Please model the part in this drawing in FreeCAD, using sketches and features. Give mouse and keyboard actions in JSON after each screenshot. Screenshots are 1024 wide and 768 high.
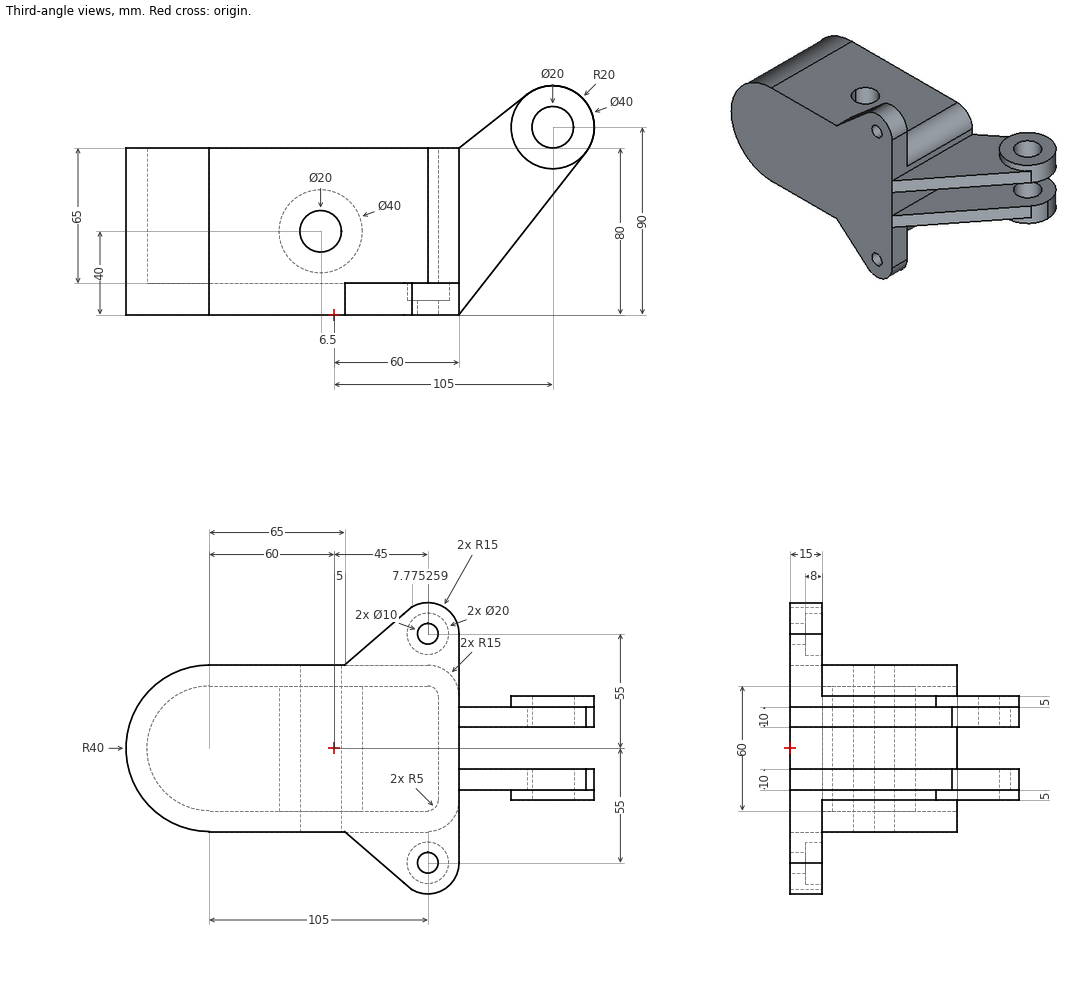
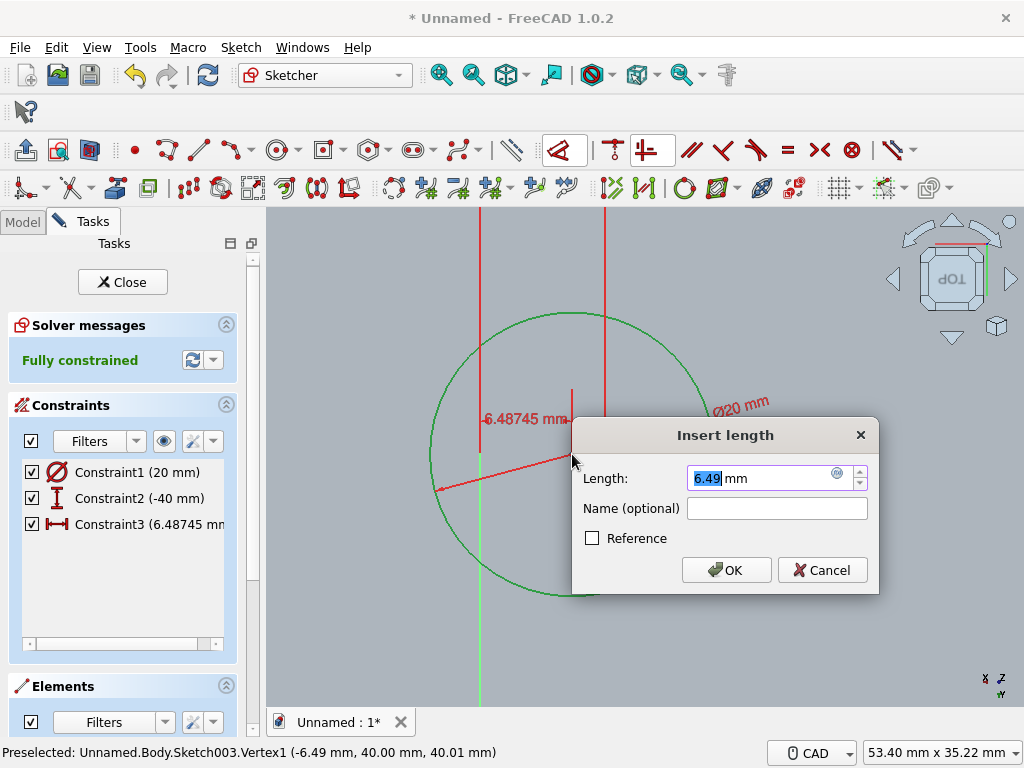
{"action": "type", "text": "6.5"}
{"action": "key", "text": "Return"}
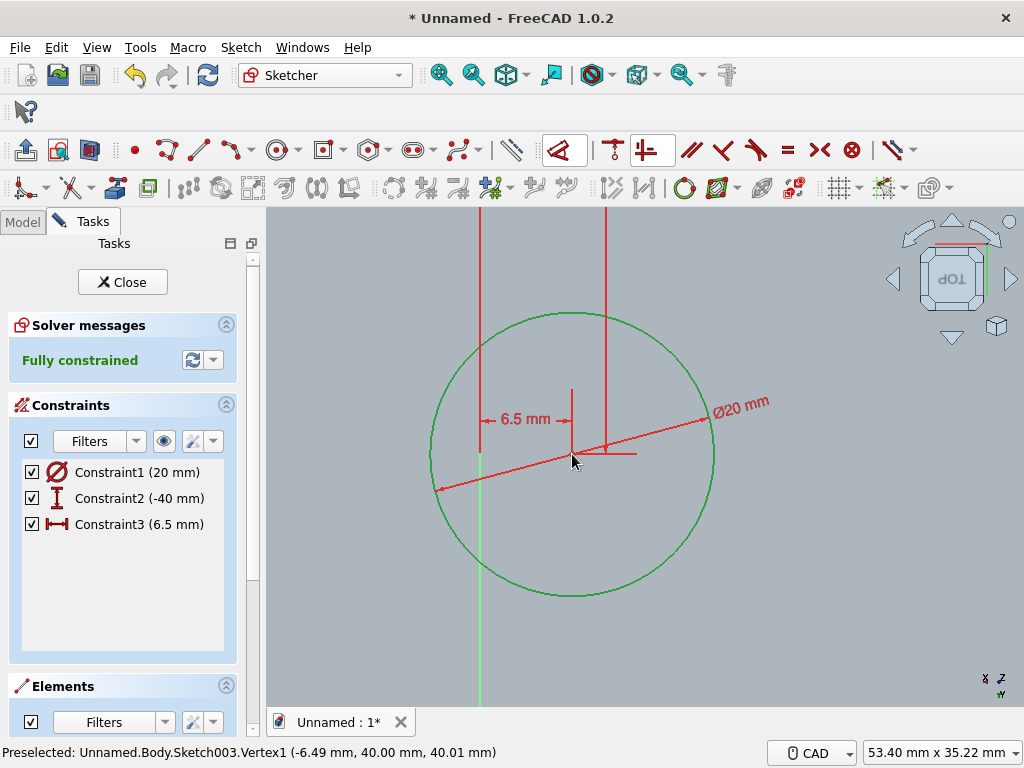
{"action": "left_click", "coordinate": [123, 282]}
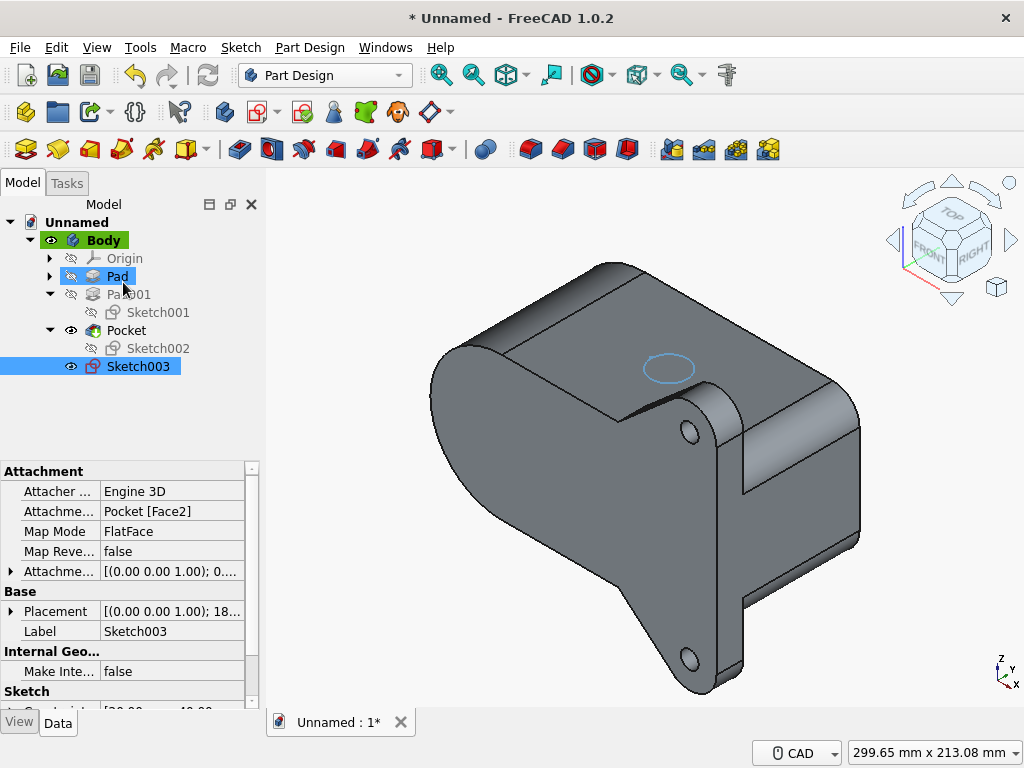
{"action": "left_click", "coordinate": [240, 150]}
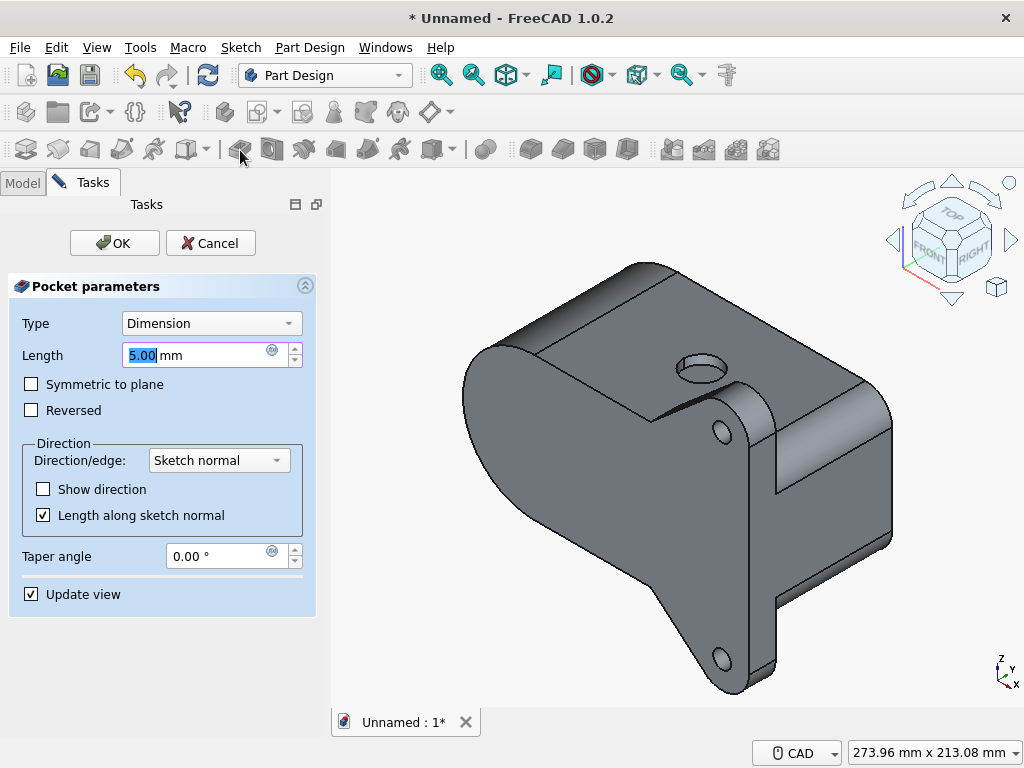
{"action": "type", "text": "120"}
{"action": "key", "text": "Tab"}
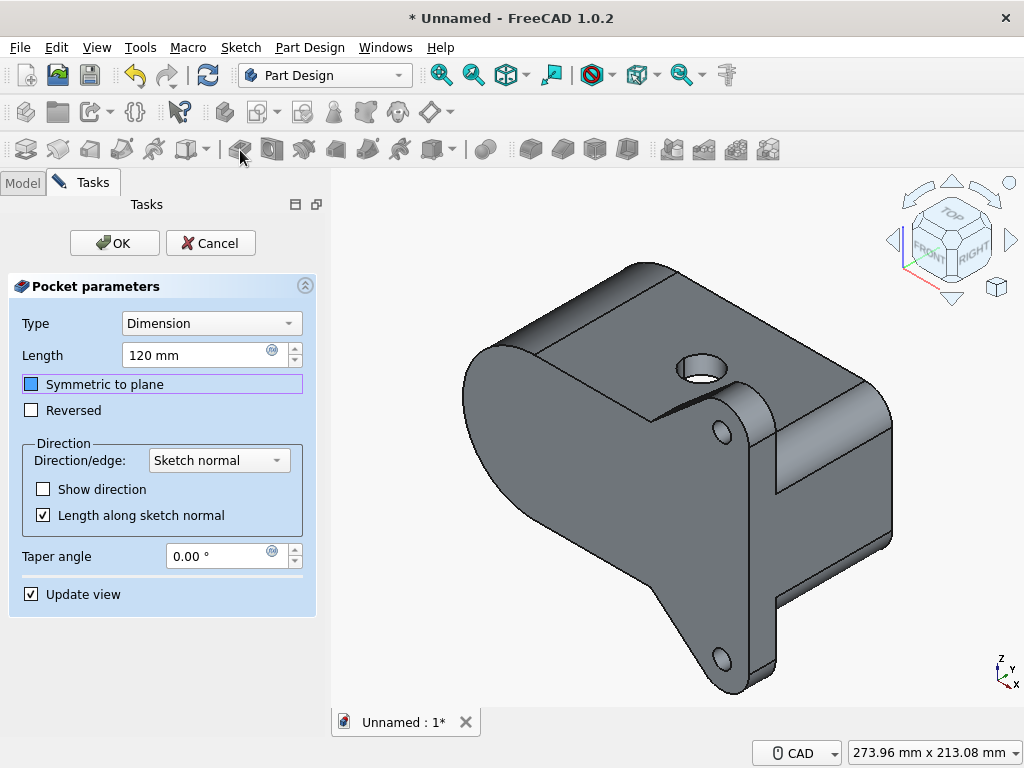
{"action": "left_click", "coordinate": [115, 243]}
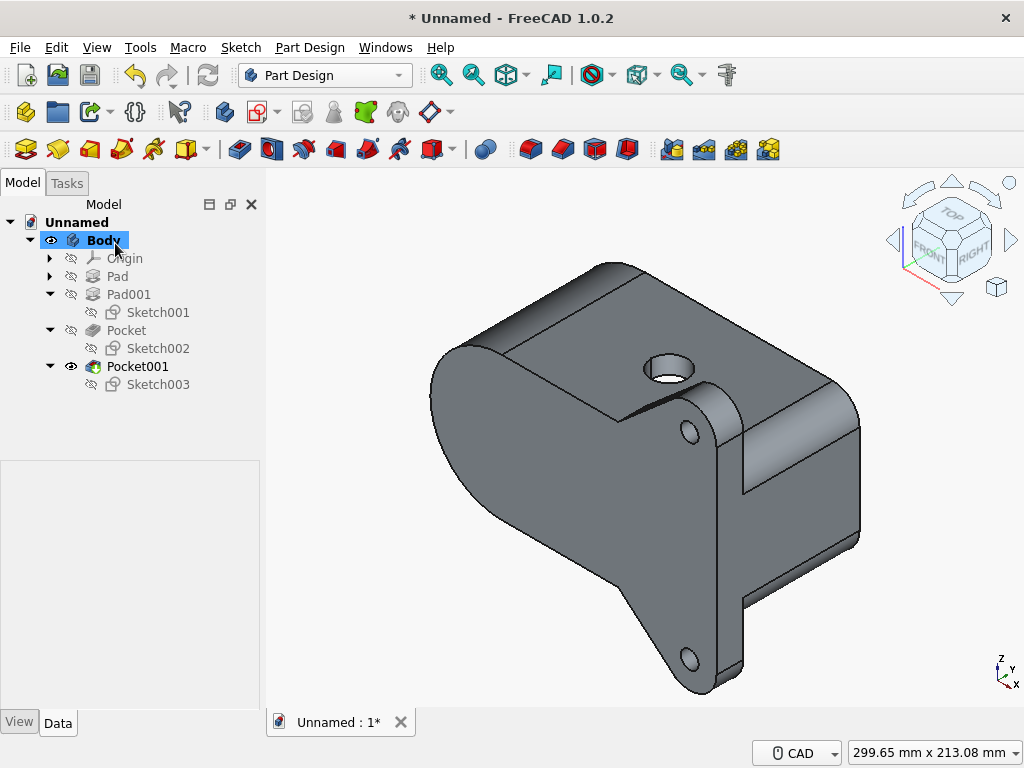
{"action": "left_click", "coordinate": [50, 258]}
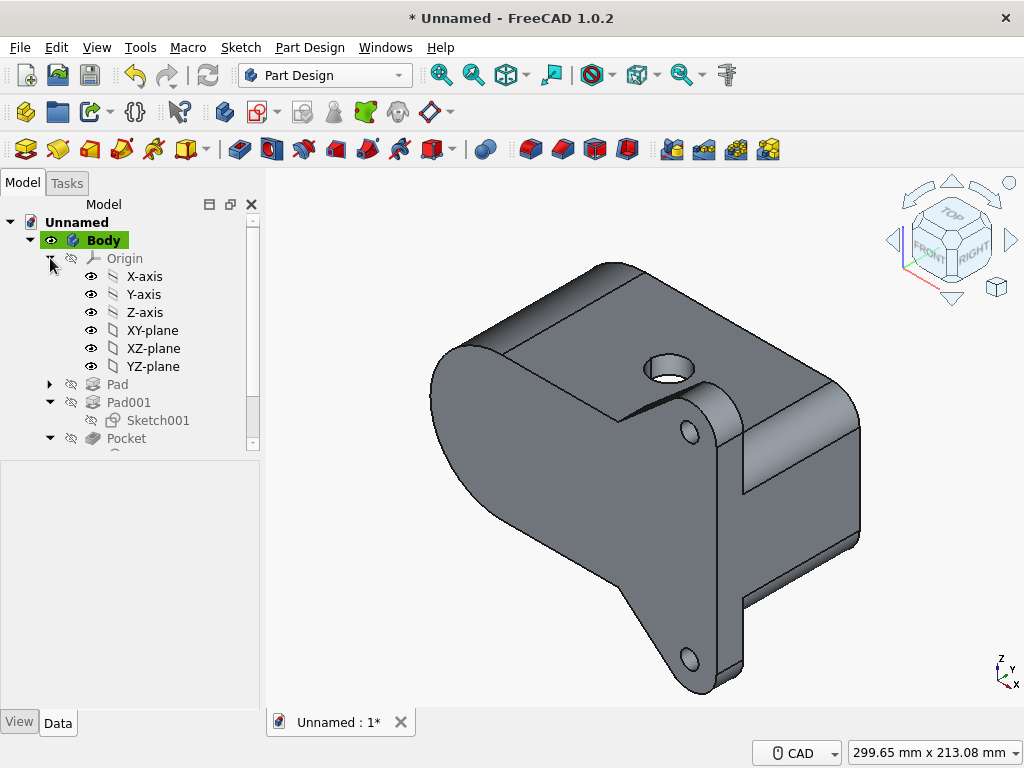
{"action": "left_click", "coordinate": [136, 330]}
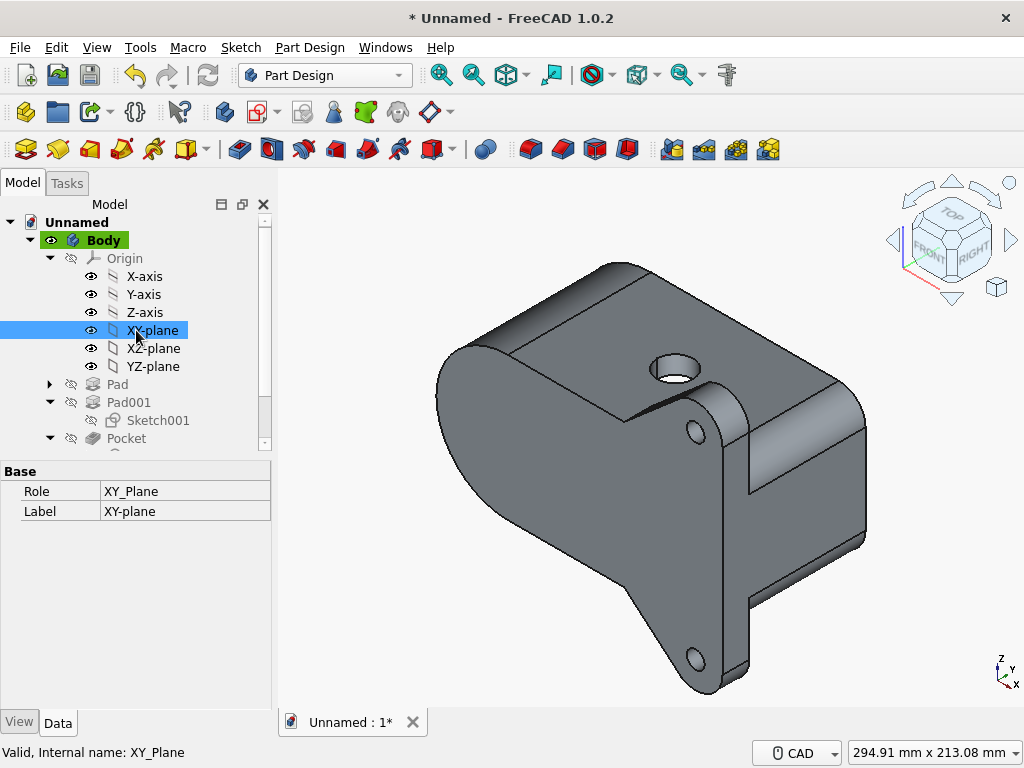
{"action": "left_click", "coordinate": [430, 112]}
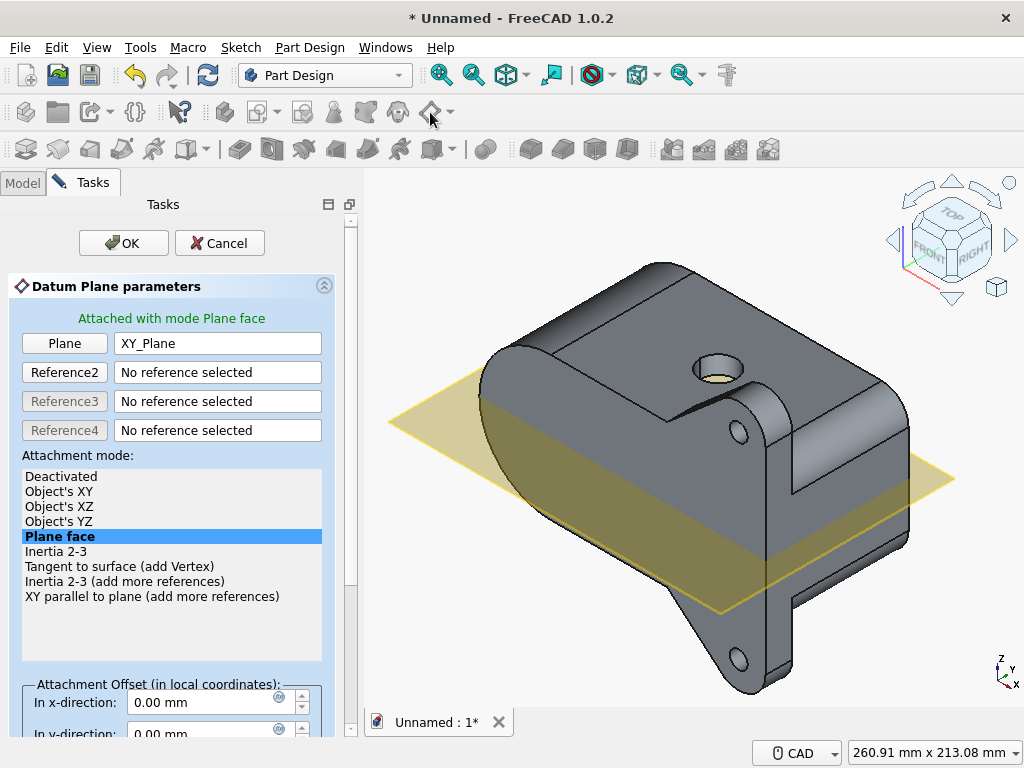
{"action": "scroll", "coordinate": [351, 475], "scroll_direction": "down", "scroll_amount": 2}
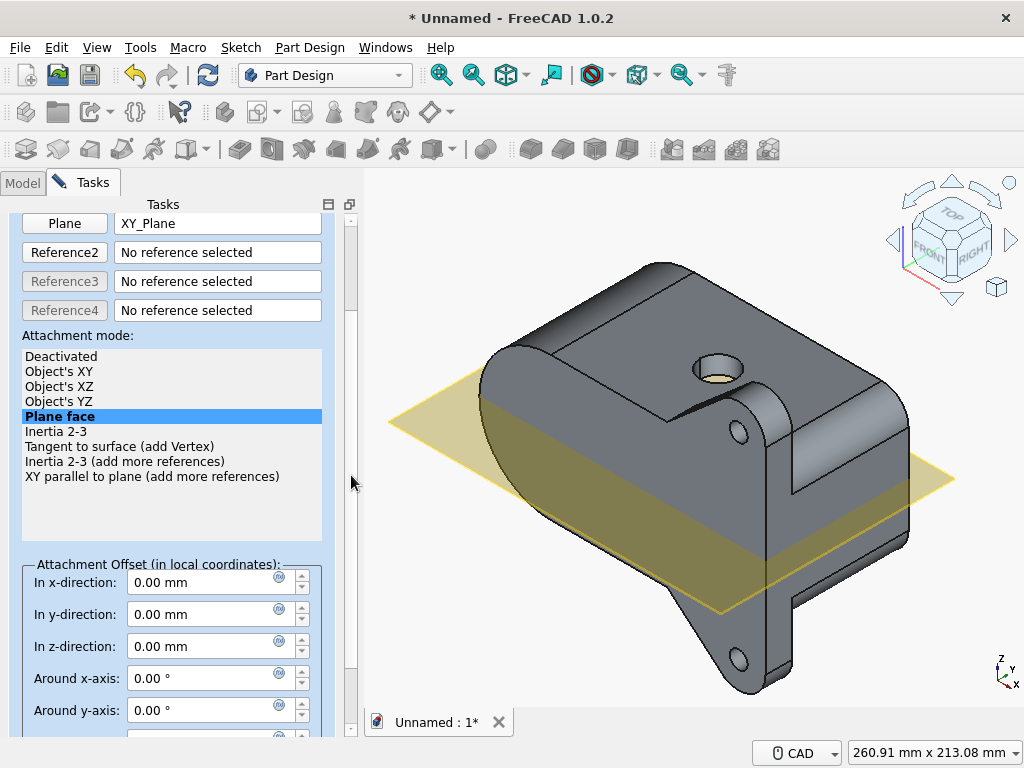
{"action": "triple_click", "coordinate": [210, 646]}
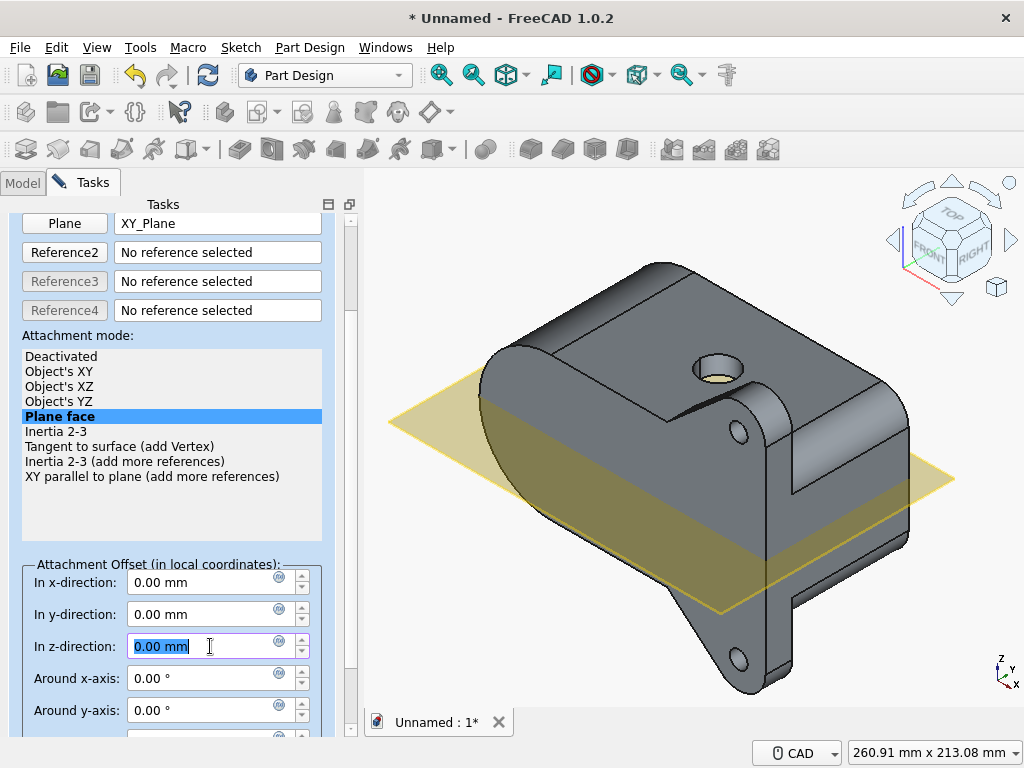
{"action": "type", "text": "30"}
{"action": "key", "text": "Tab"}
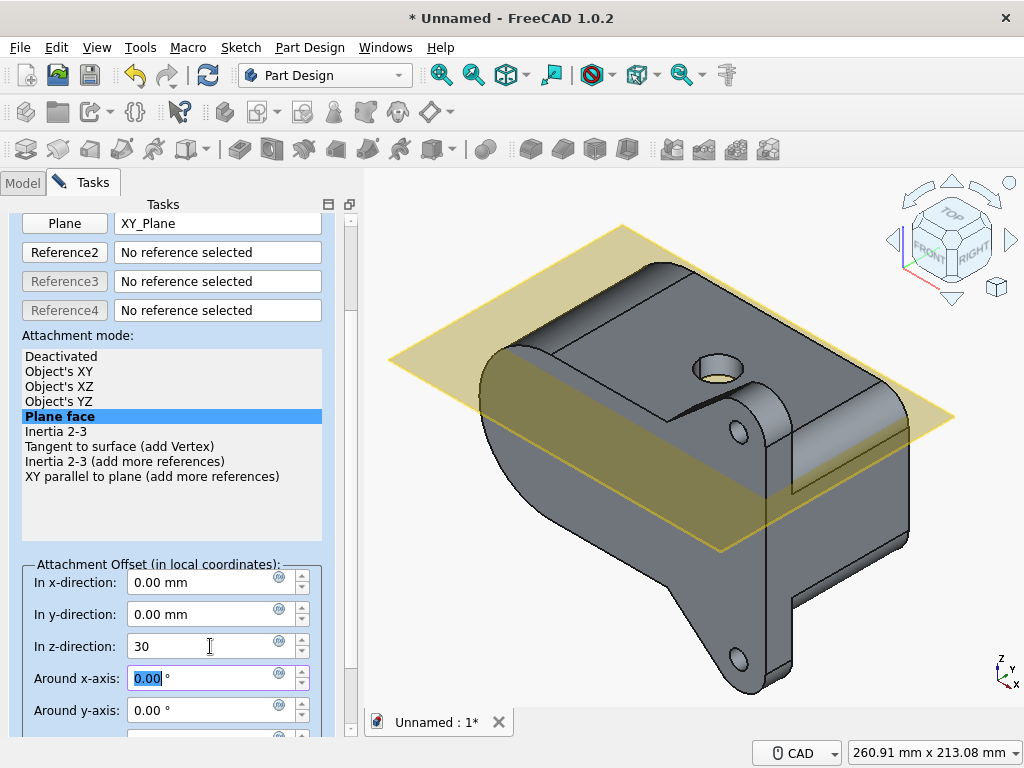
{"action": "scroll", "coordinate": [351, 475], "scroll_direction": "up", "scroll_amount": 3}